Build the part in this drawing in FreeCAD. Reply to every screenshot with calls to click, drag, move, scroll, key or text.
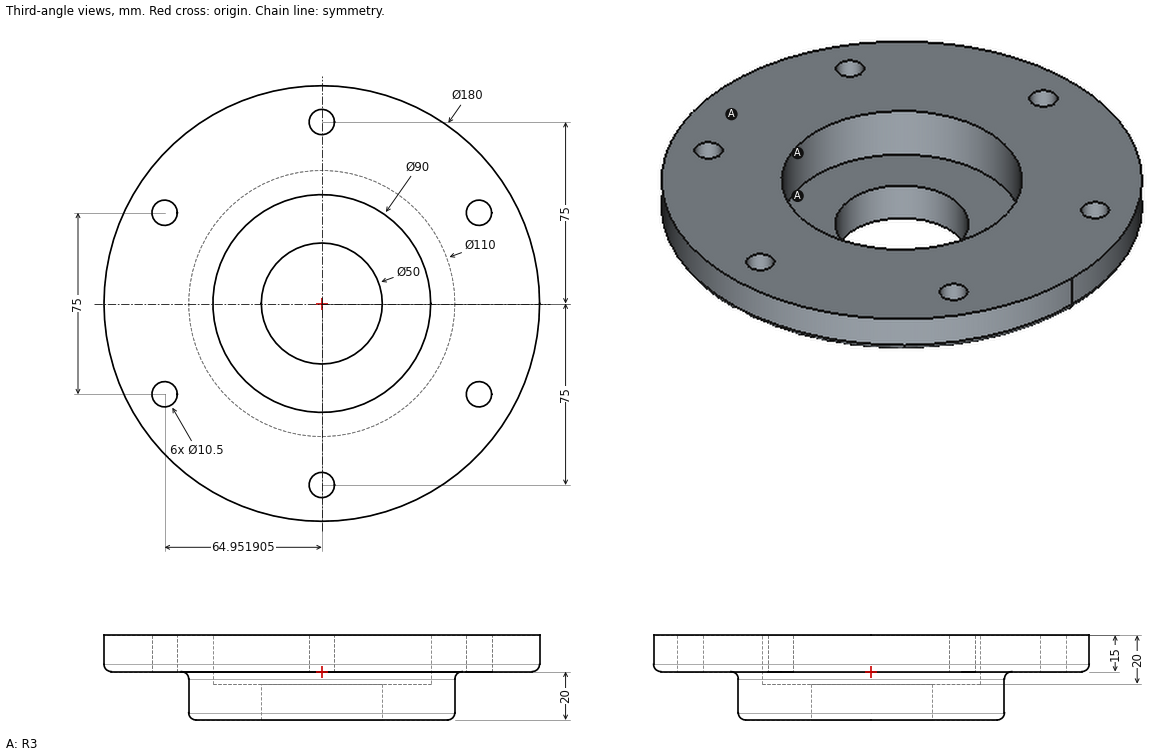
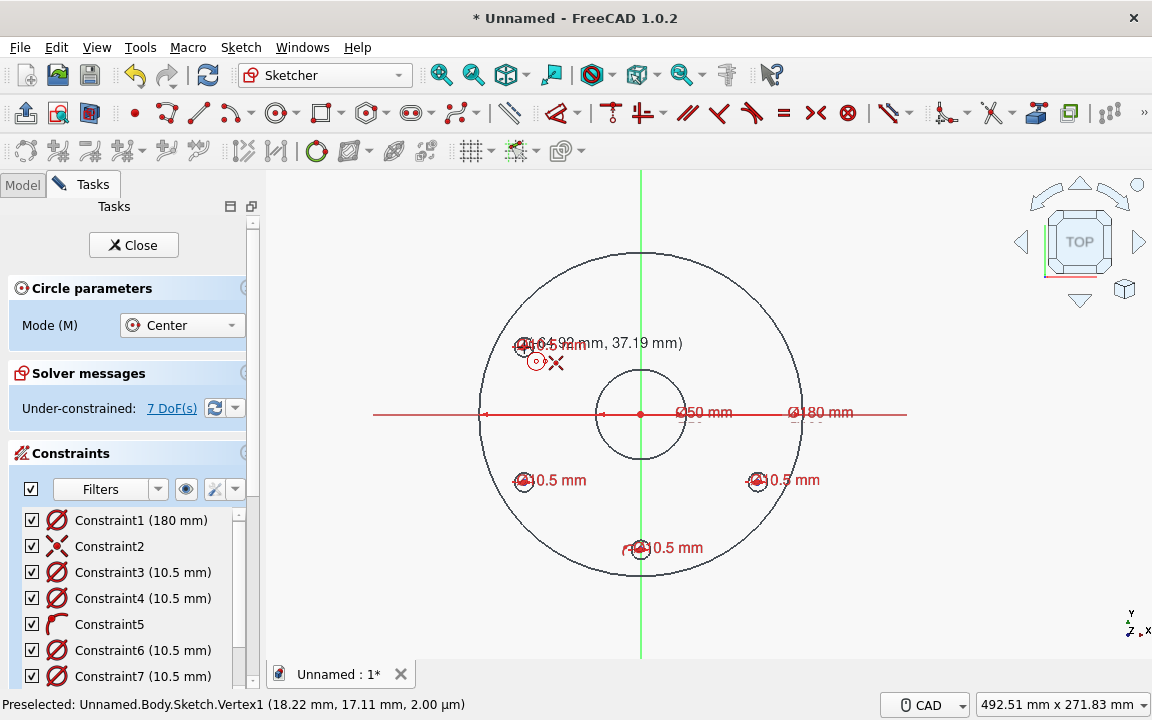
scroll(758, 347, up, 5)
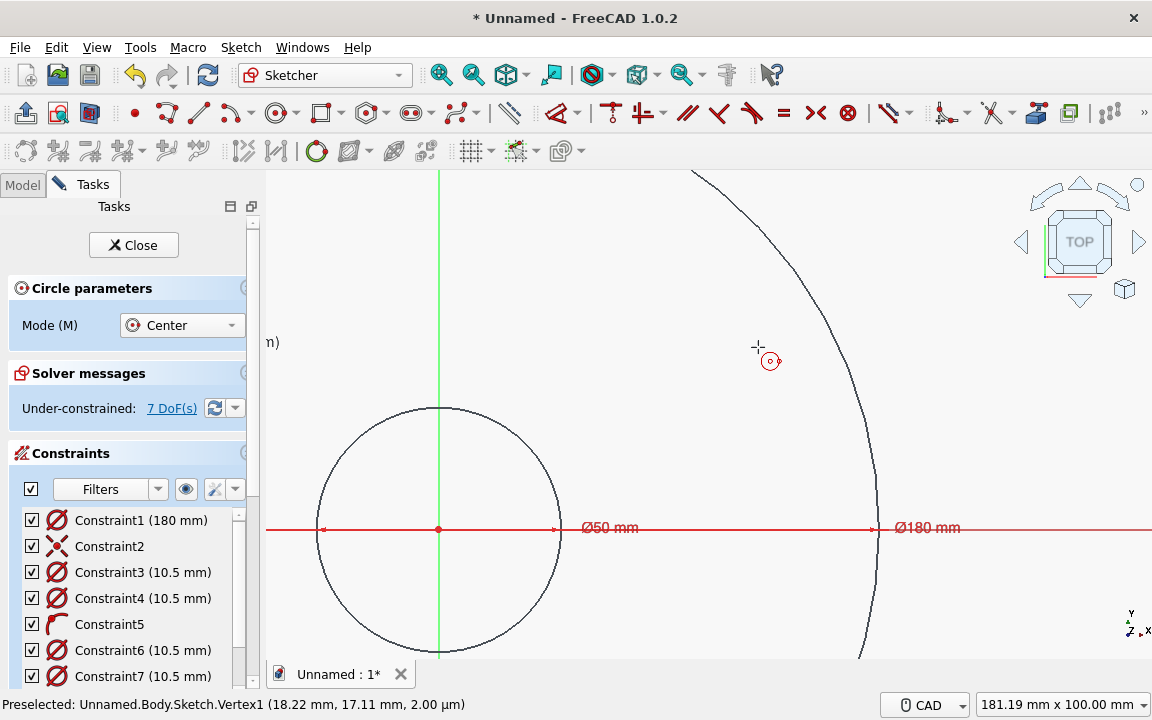
click(757, 346)
move(775, 328)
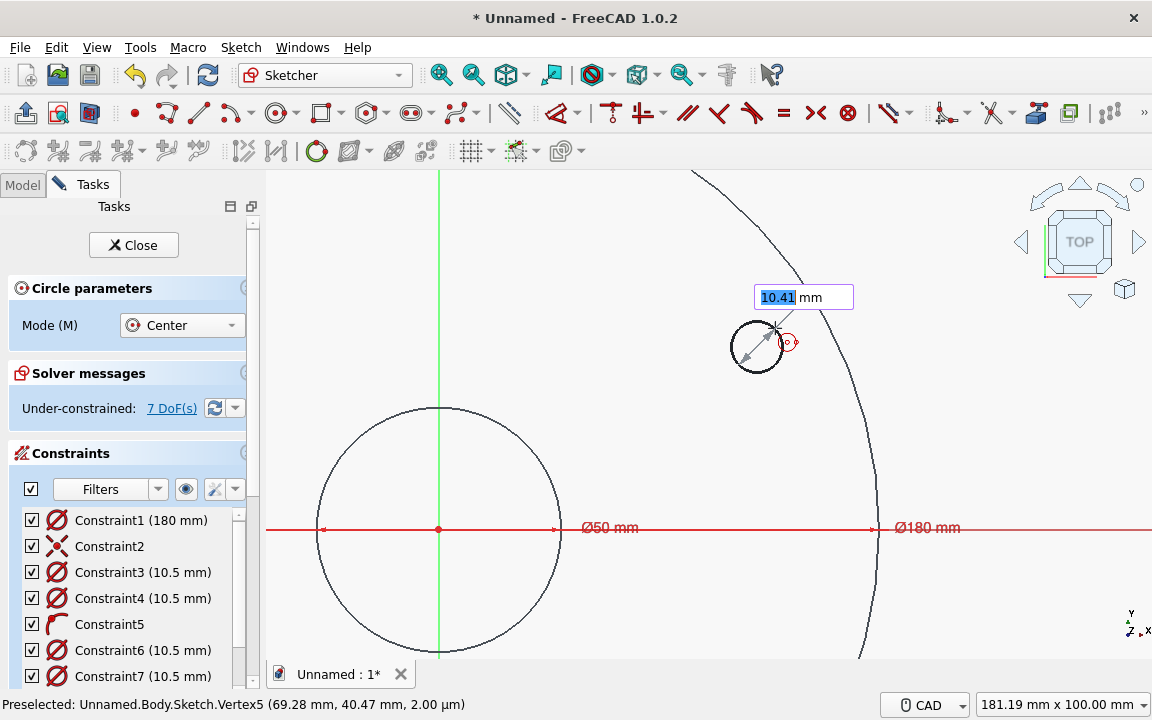
text(10.5)
key(Return)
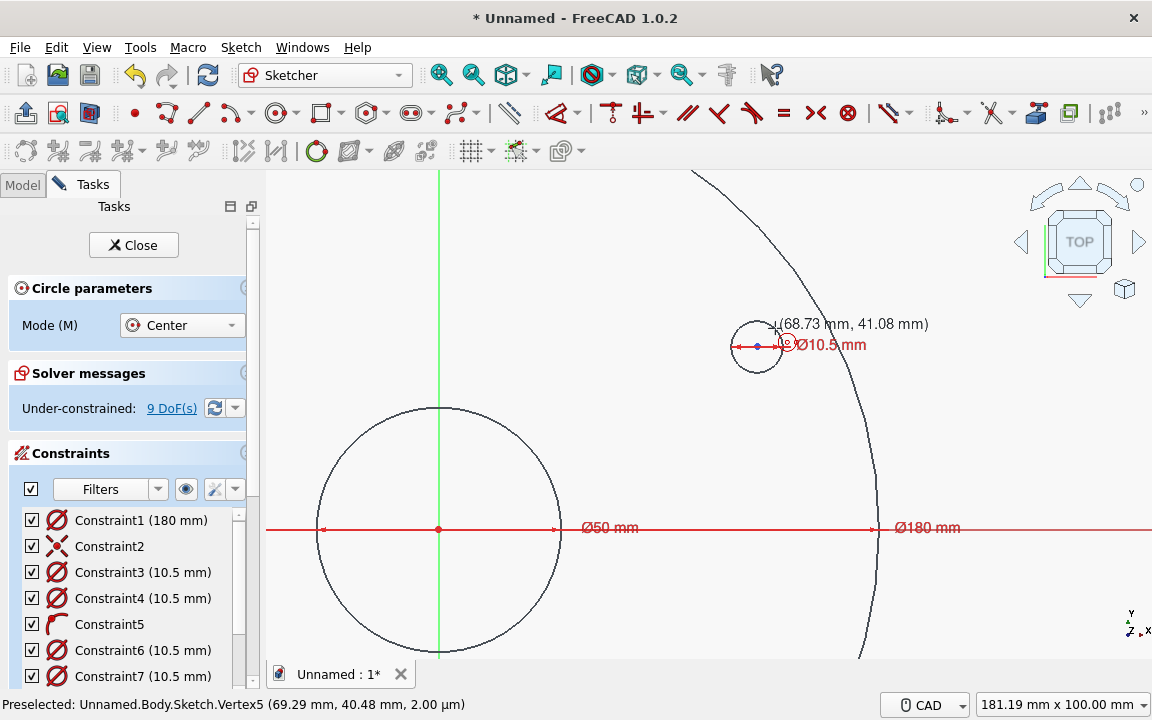
scroll(758, 347, down, 5)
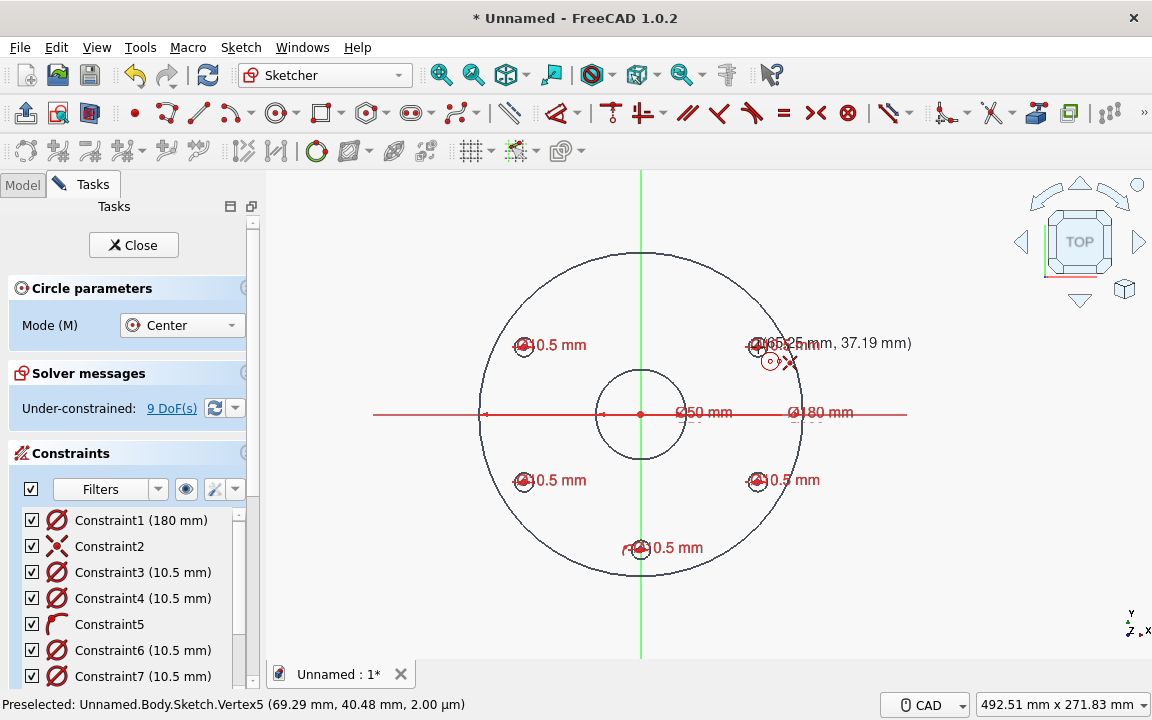
scroll(641, 280, up, 5)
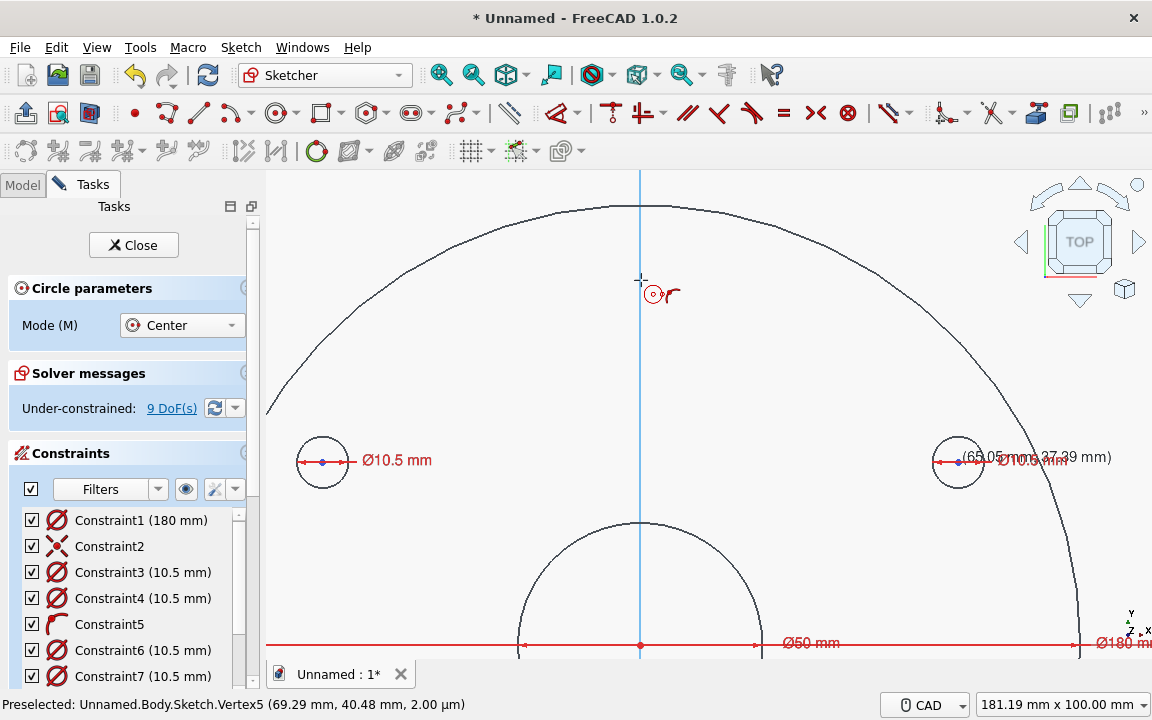
click(640, 278)
move(658, 260)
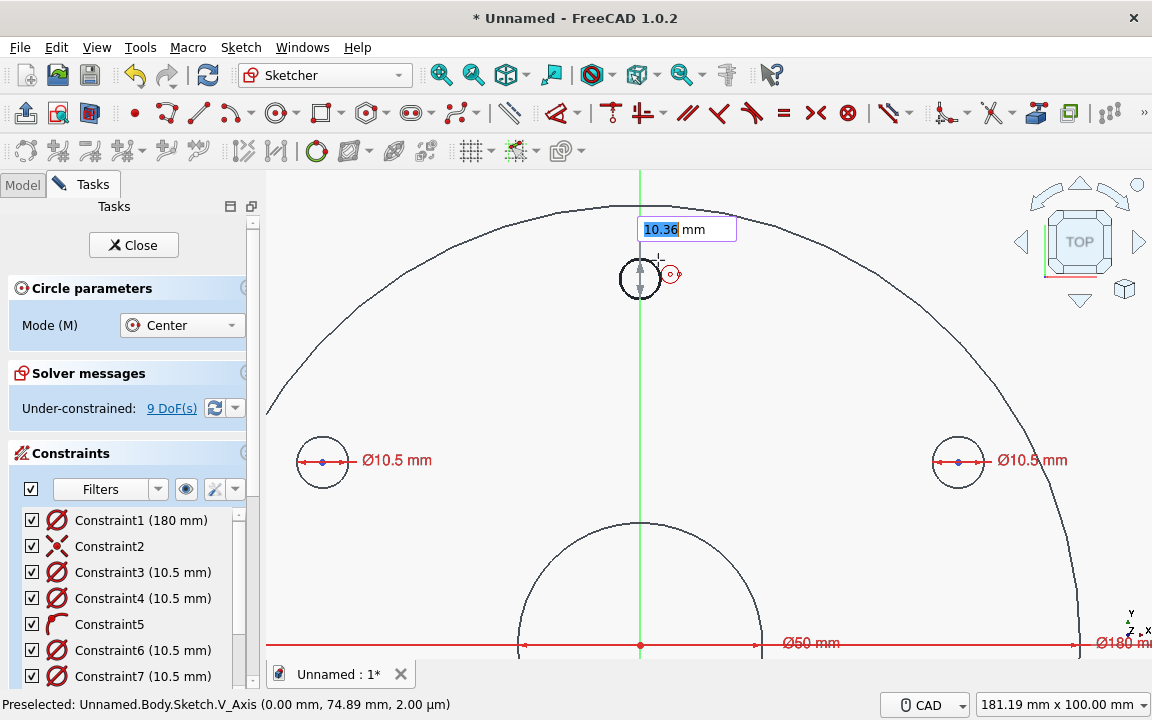
text(10.5)
key(Return)
key(Escape)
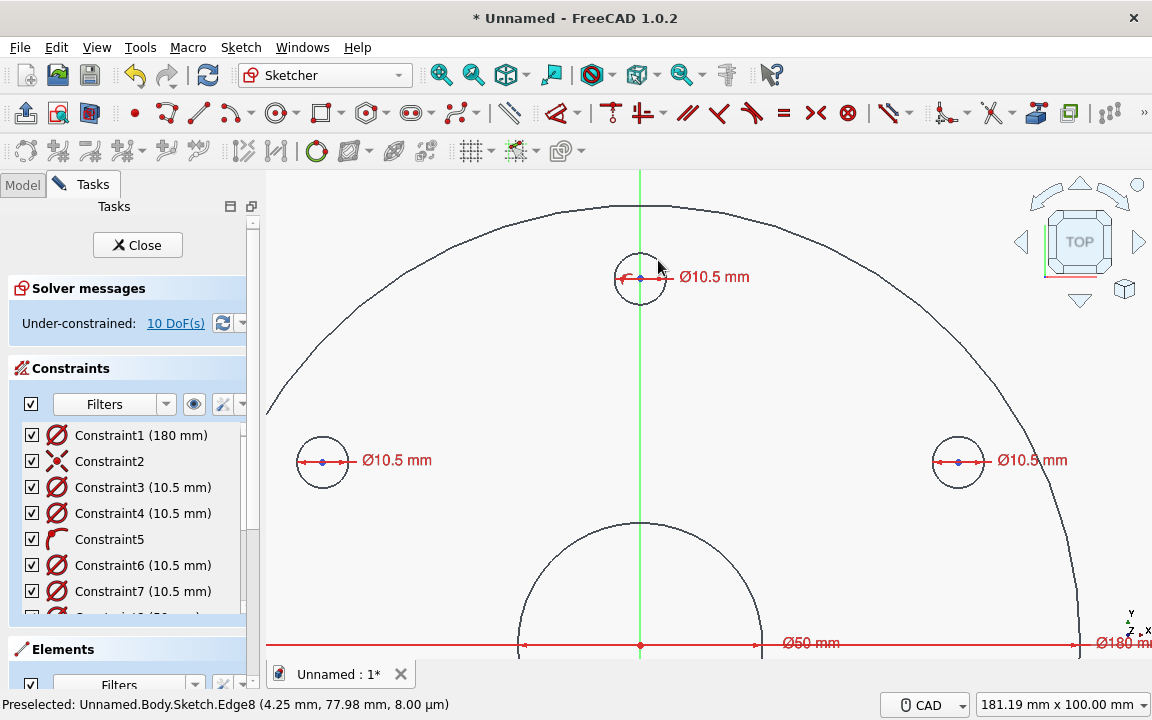
scroll(641, 280, down, 5)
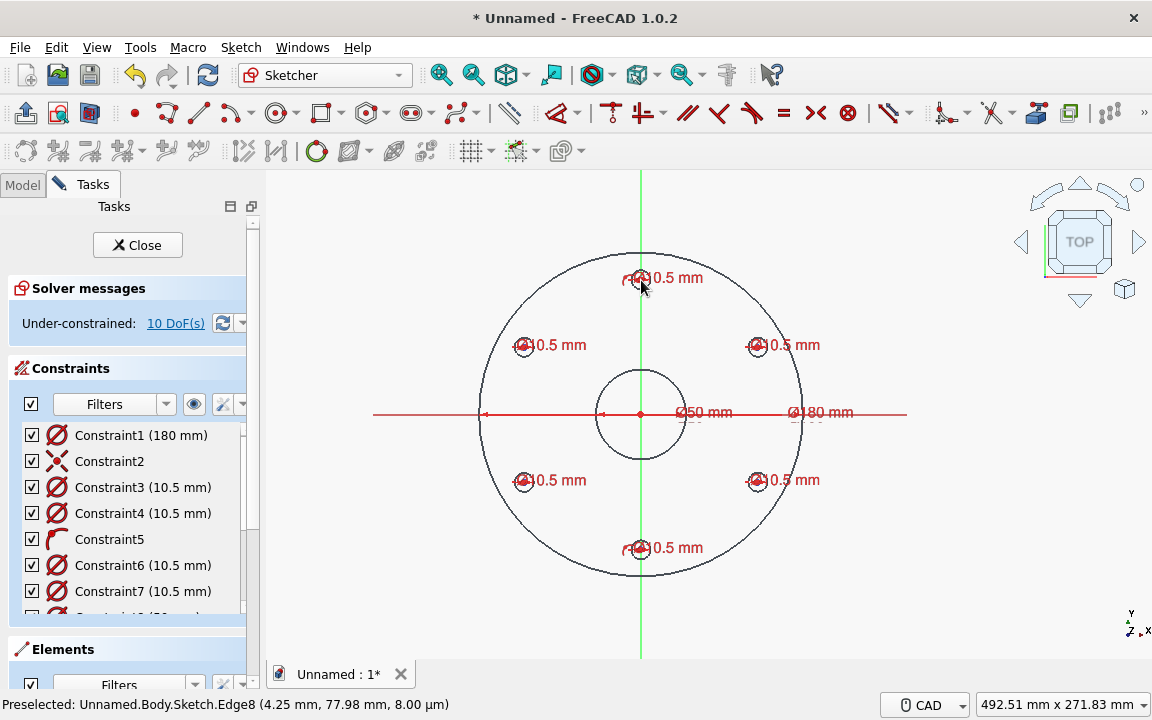
click(524, 482)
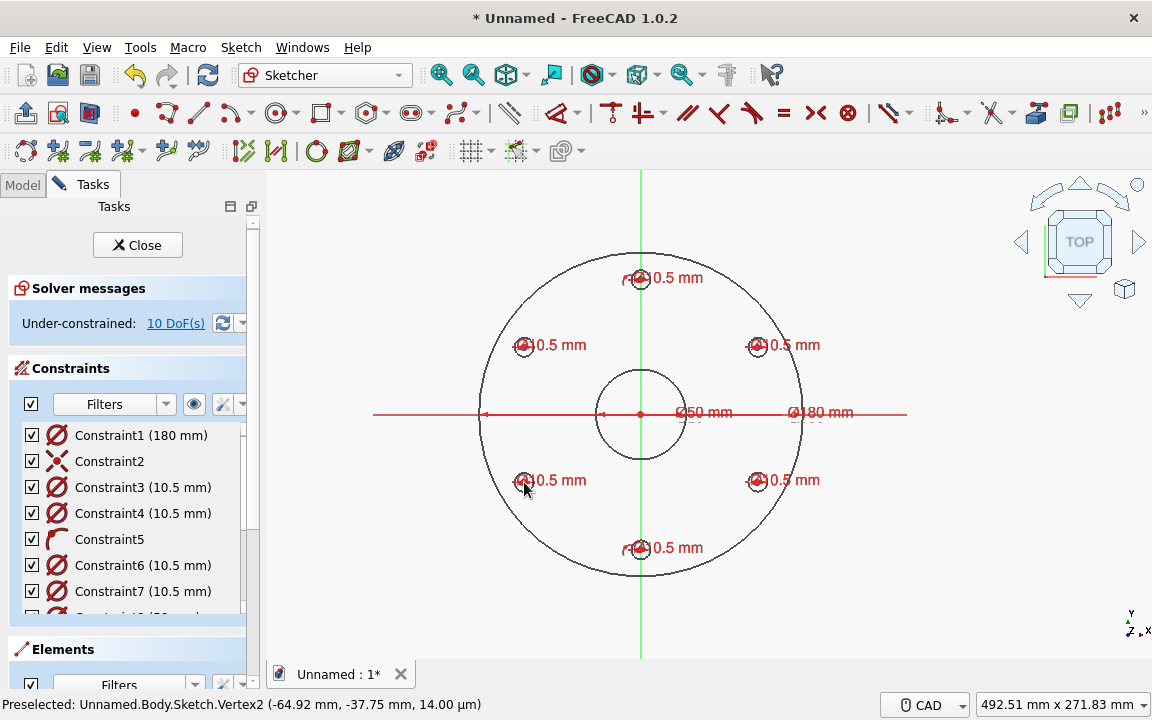
click(758, 482)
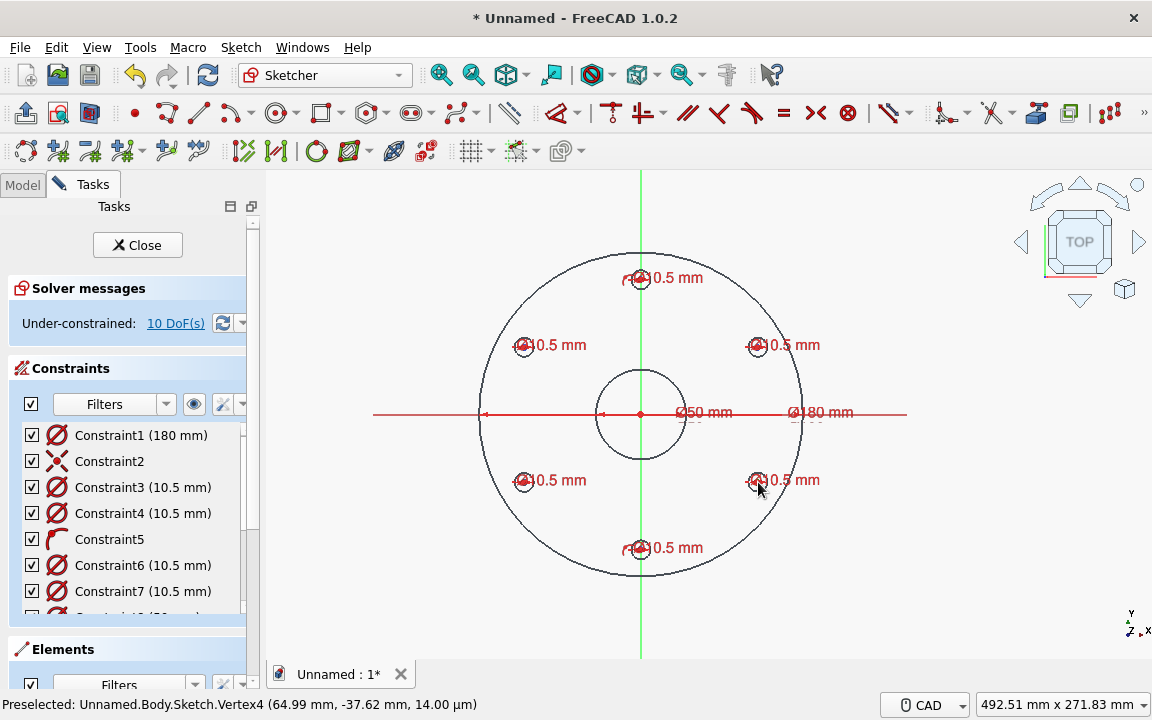
click(641, 507)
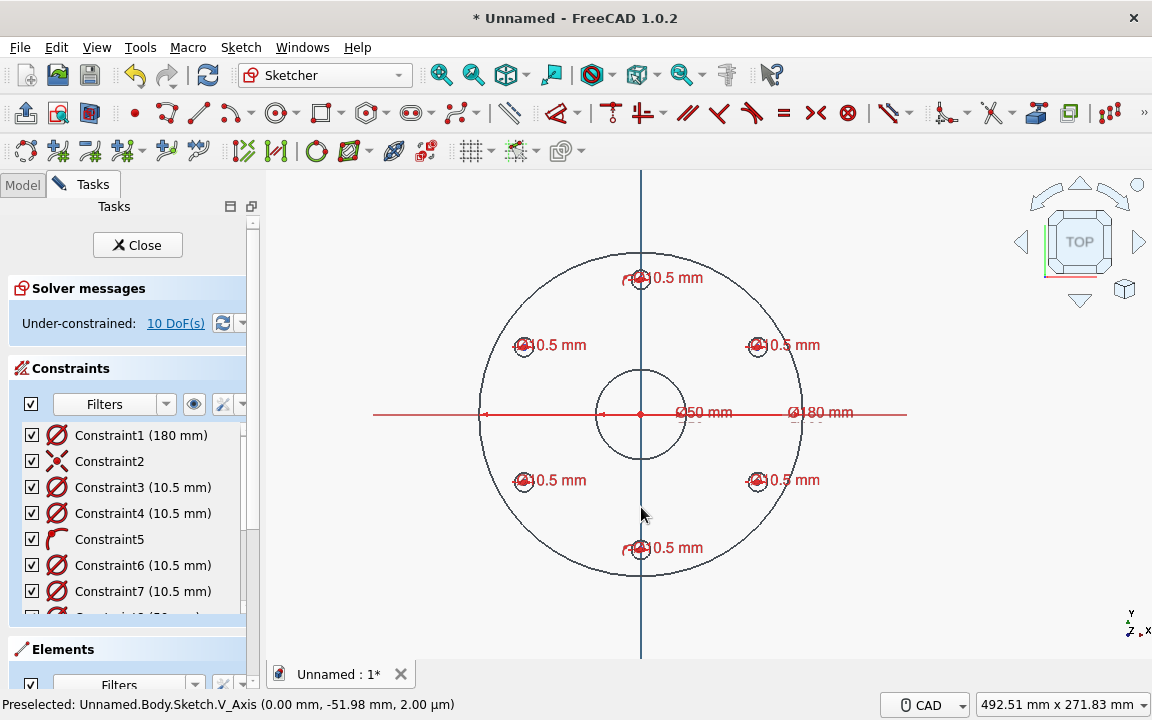
key(s)